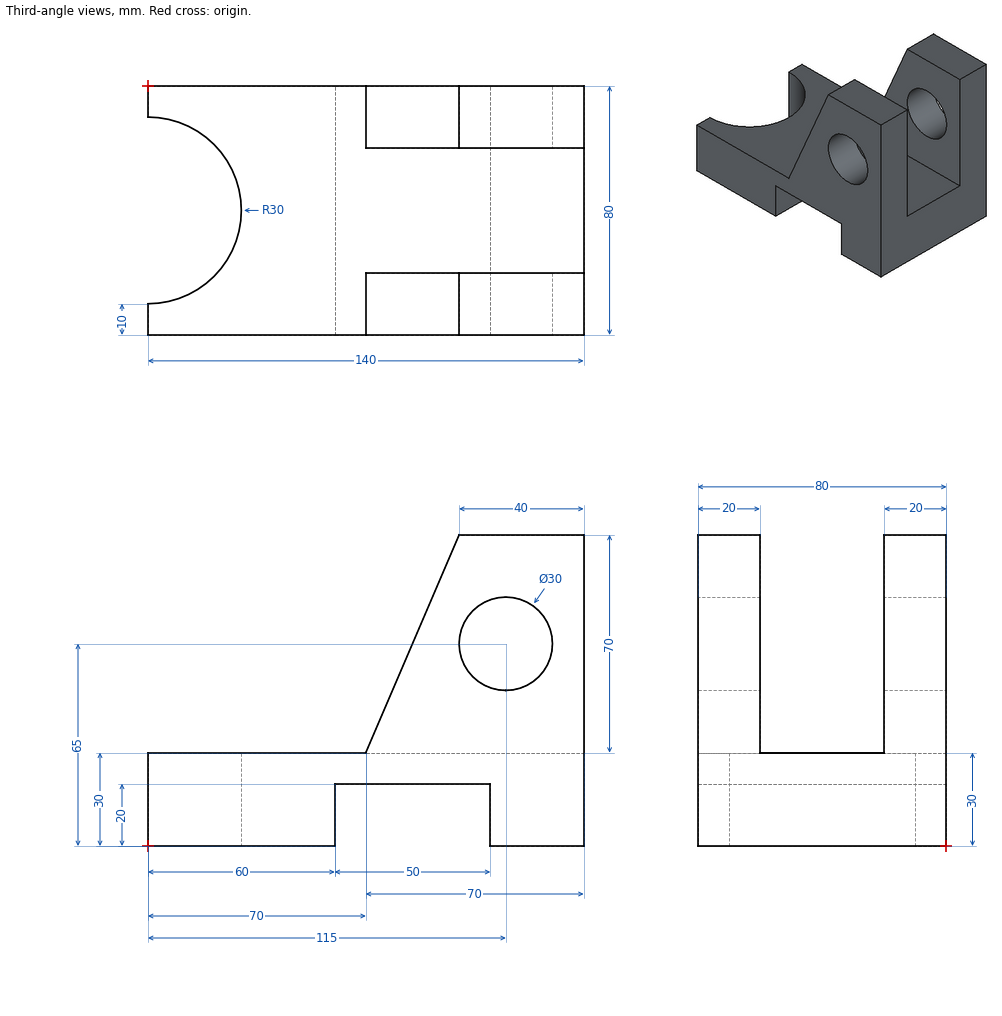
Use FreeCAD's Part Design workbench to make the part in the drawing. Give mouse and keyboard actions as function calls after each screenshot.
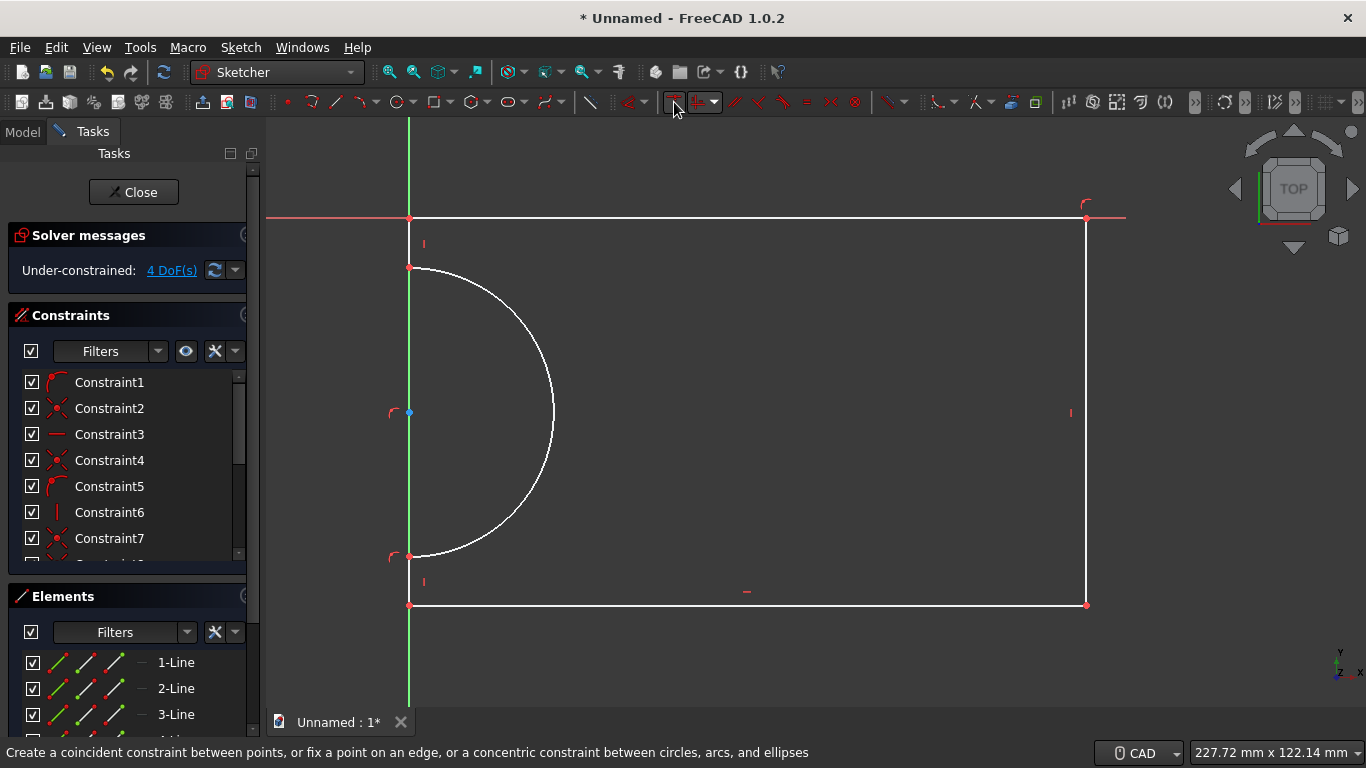
click(628, 102)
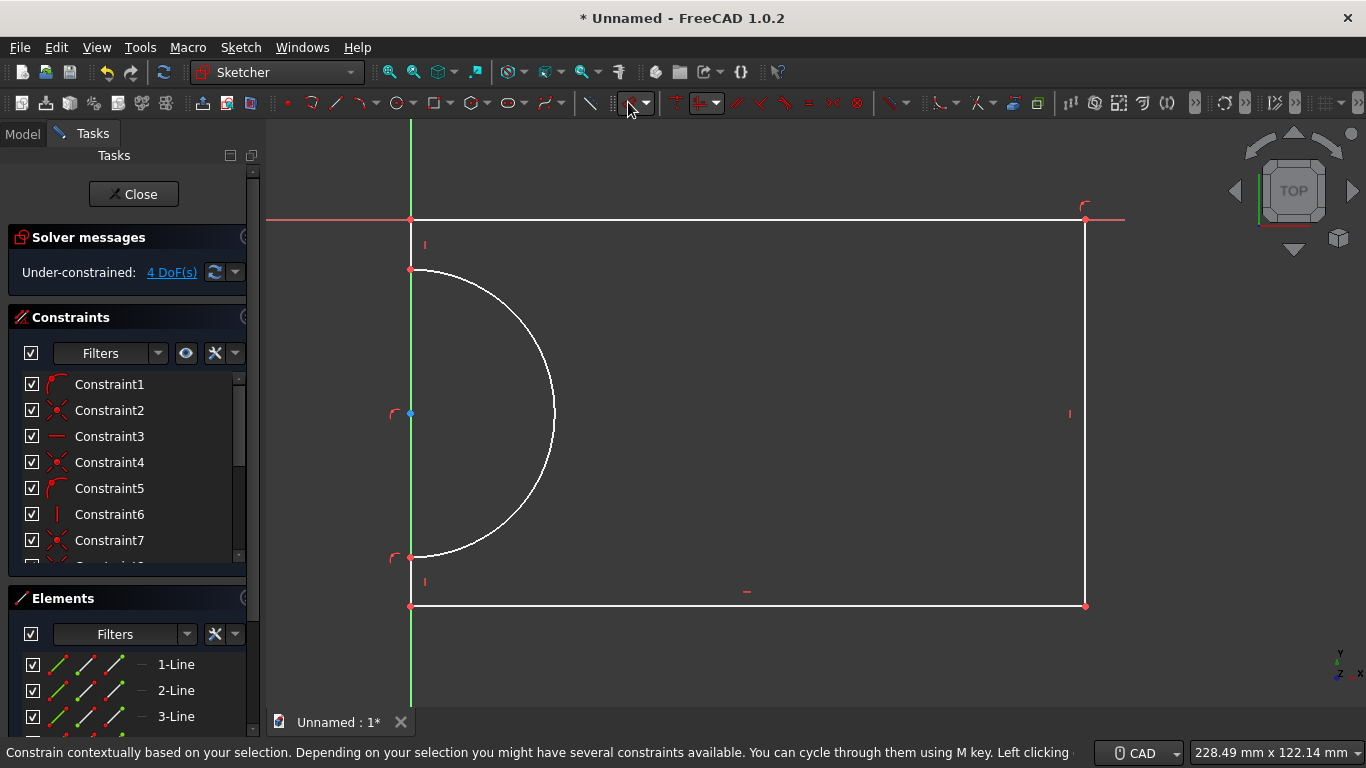
click(527, 498)
click(553, 517)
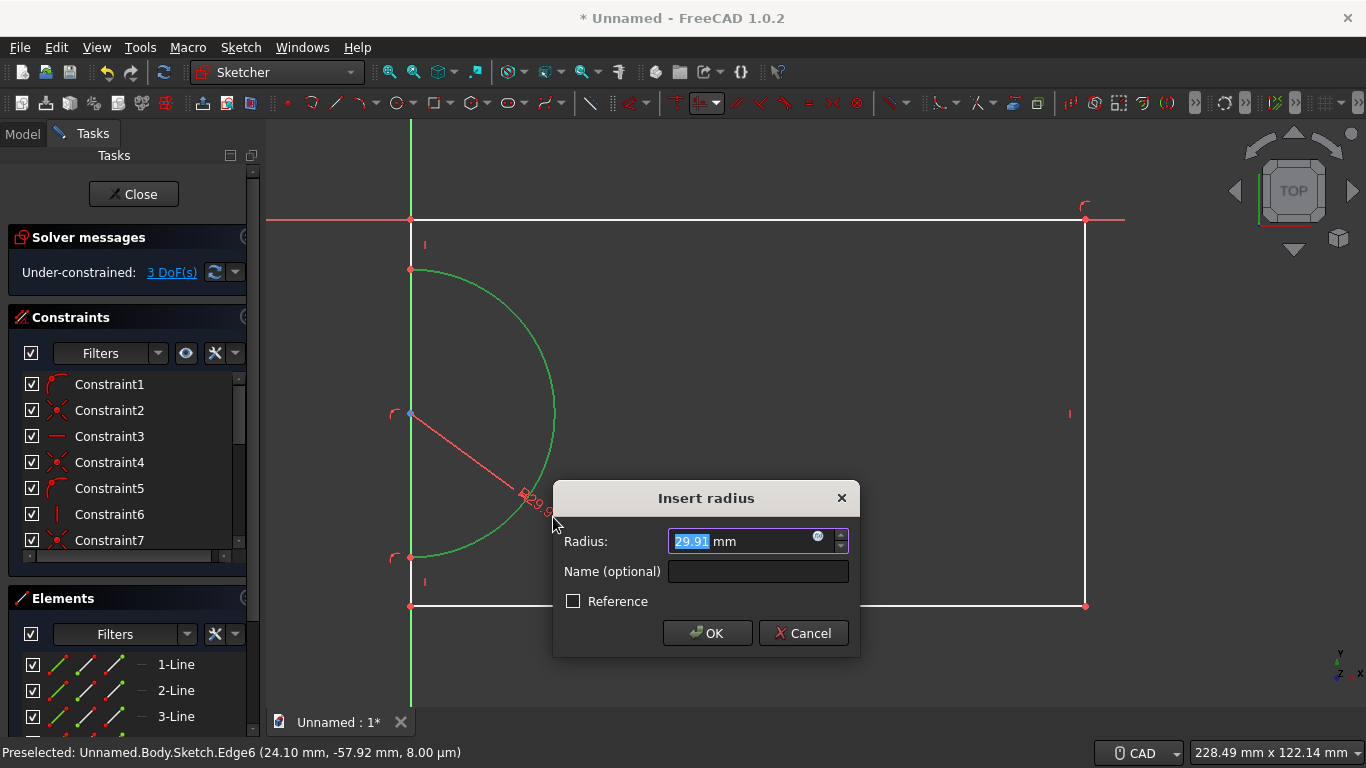
text(30)
key(Return)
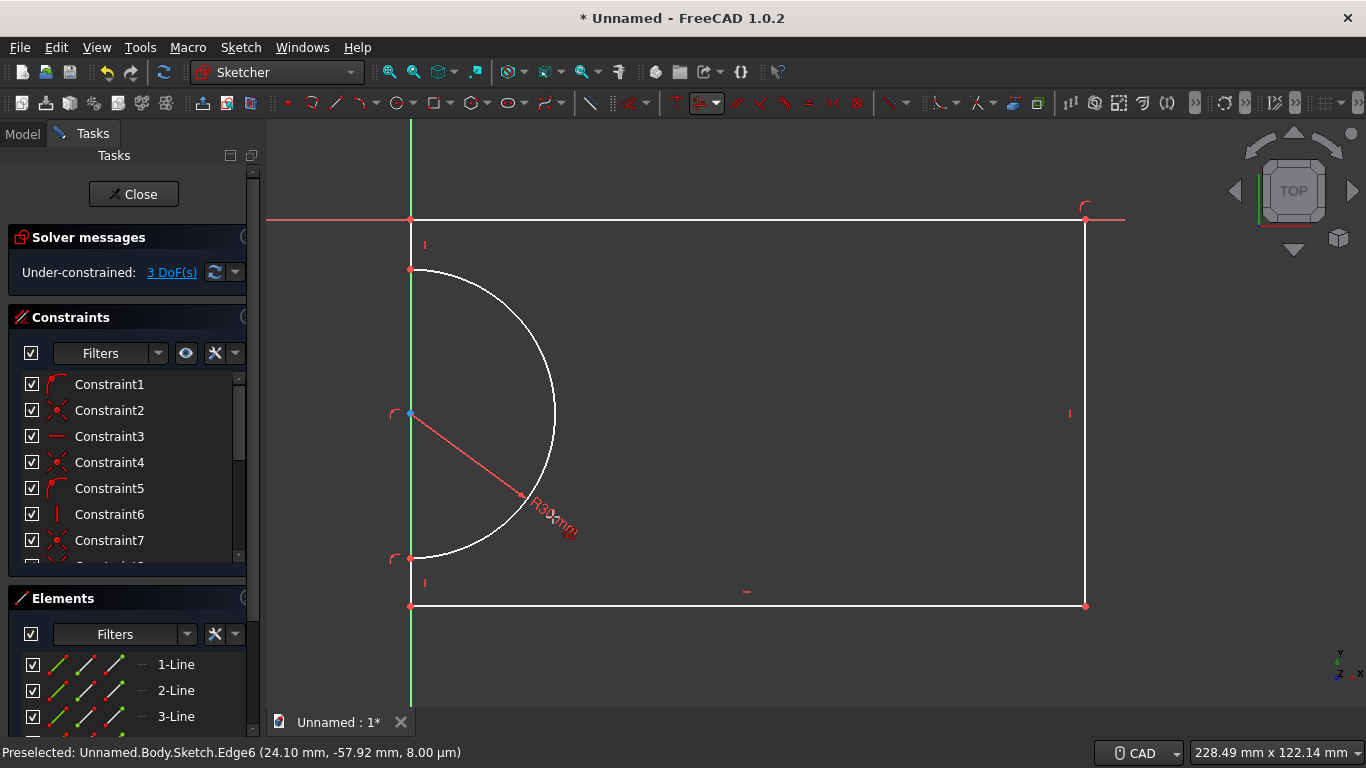
click(411, 573)
click(377, 582)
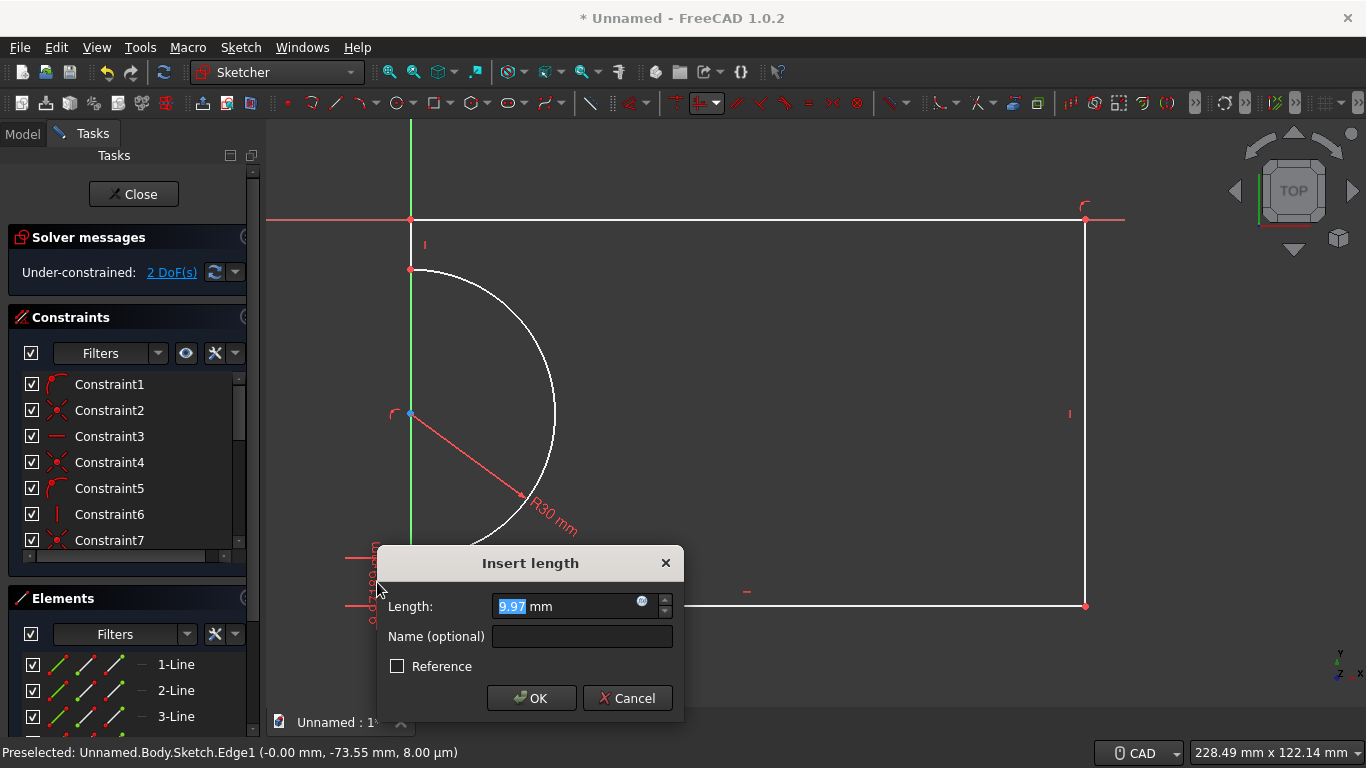
text(10)
key(Return)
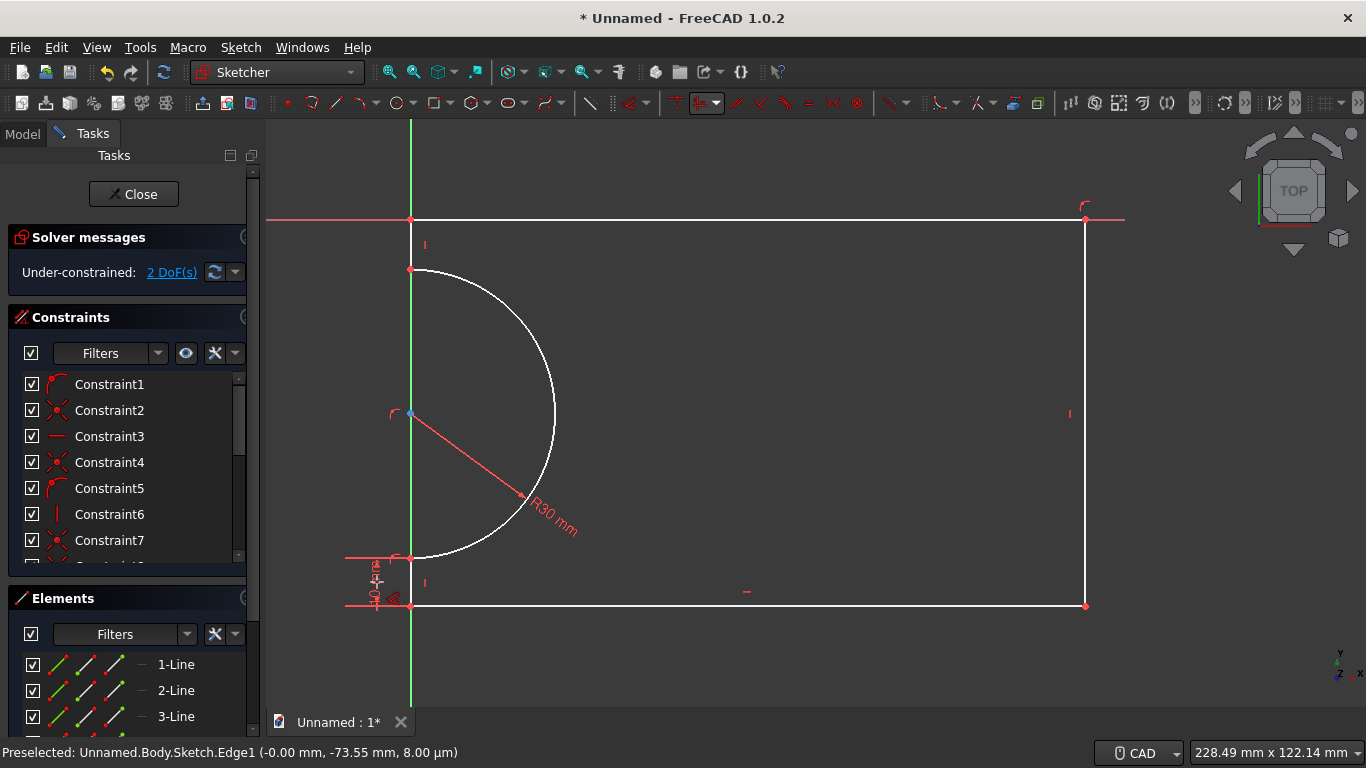
click(1085, 491)
click(1119, 413)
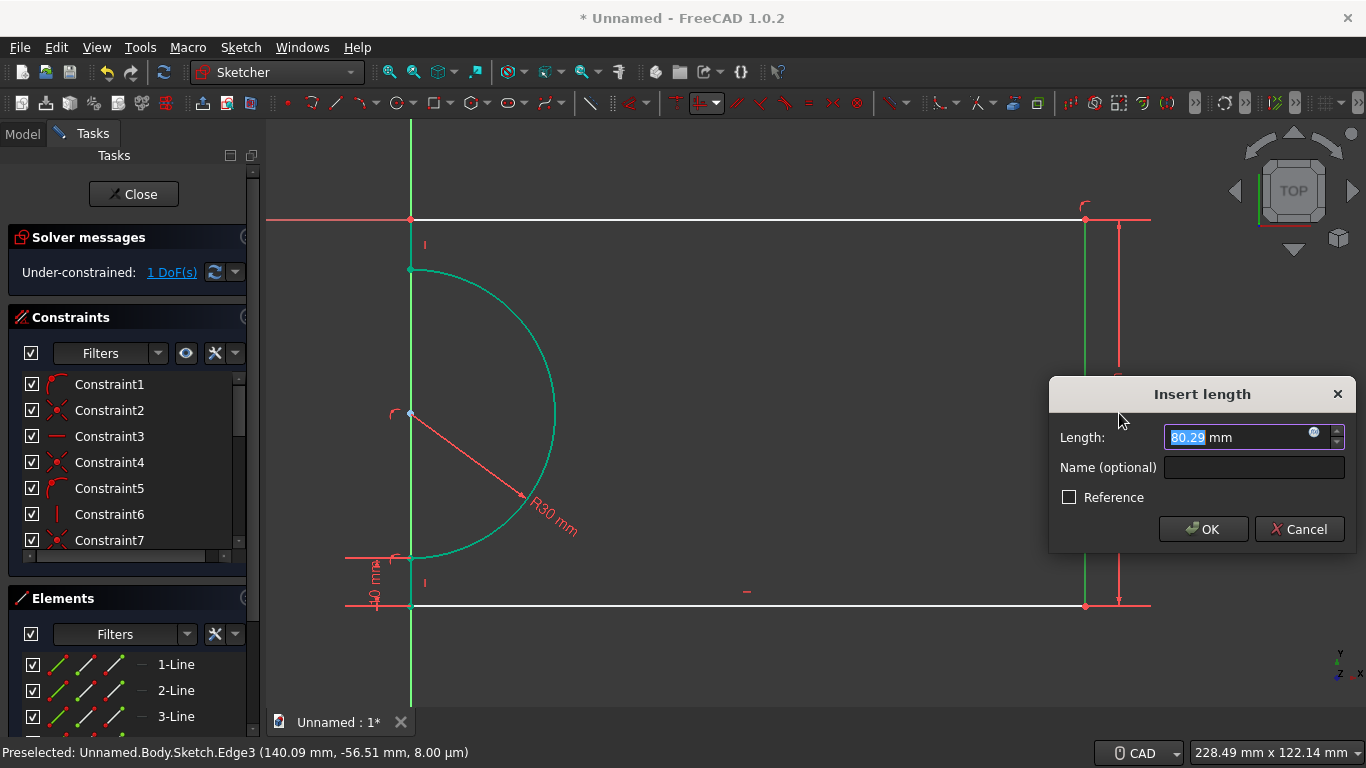
text(80)
key(Return)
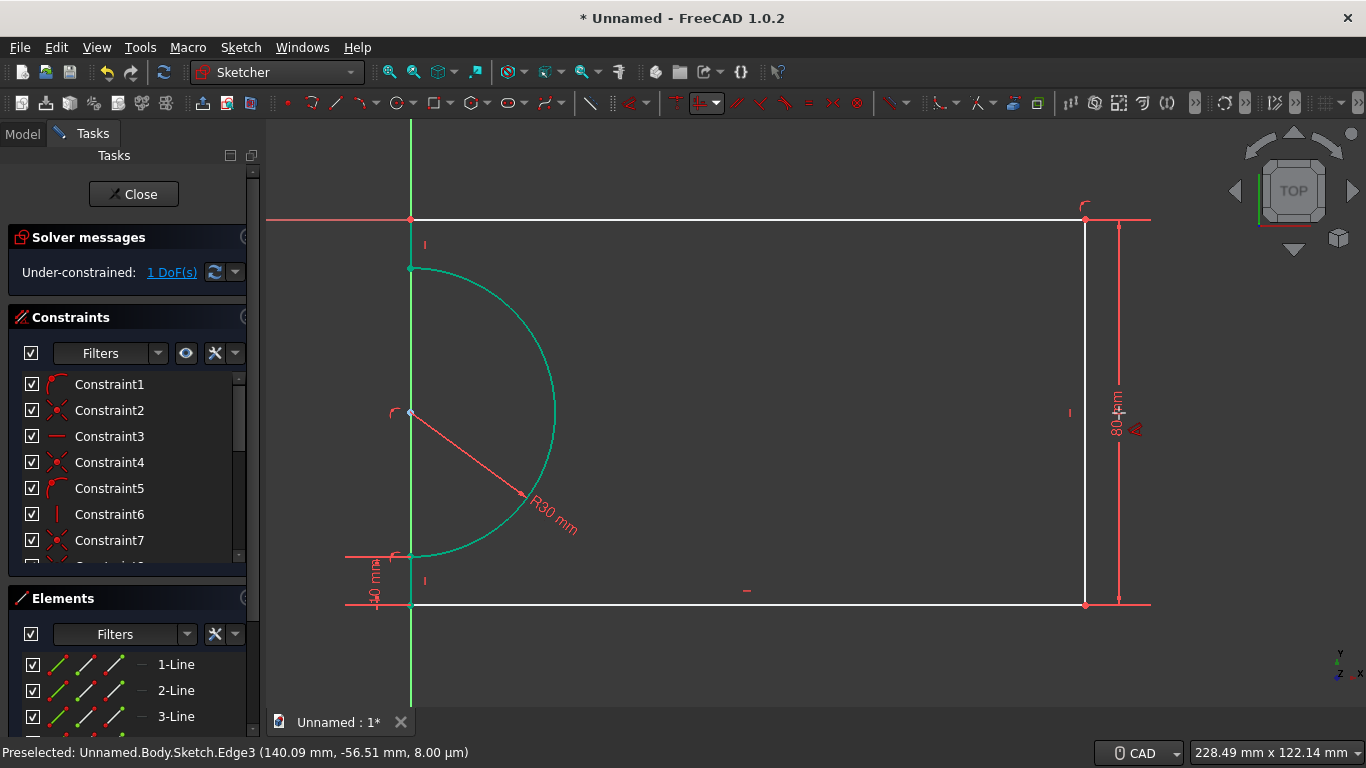
click(613, 605)
click(748, 639)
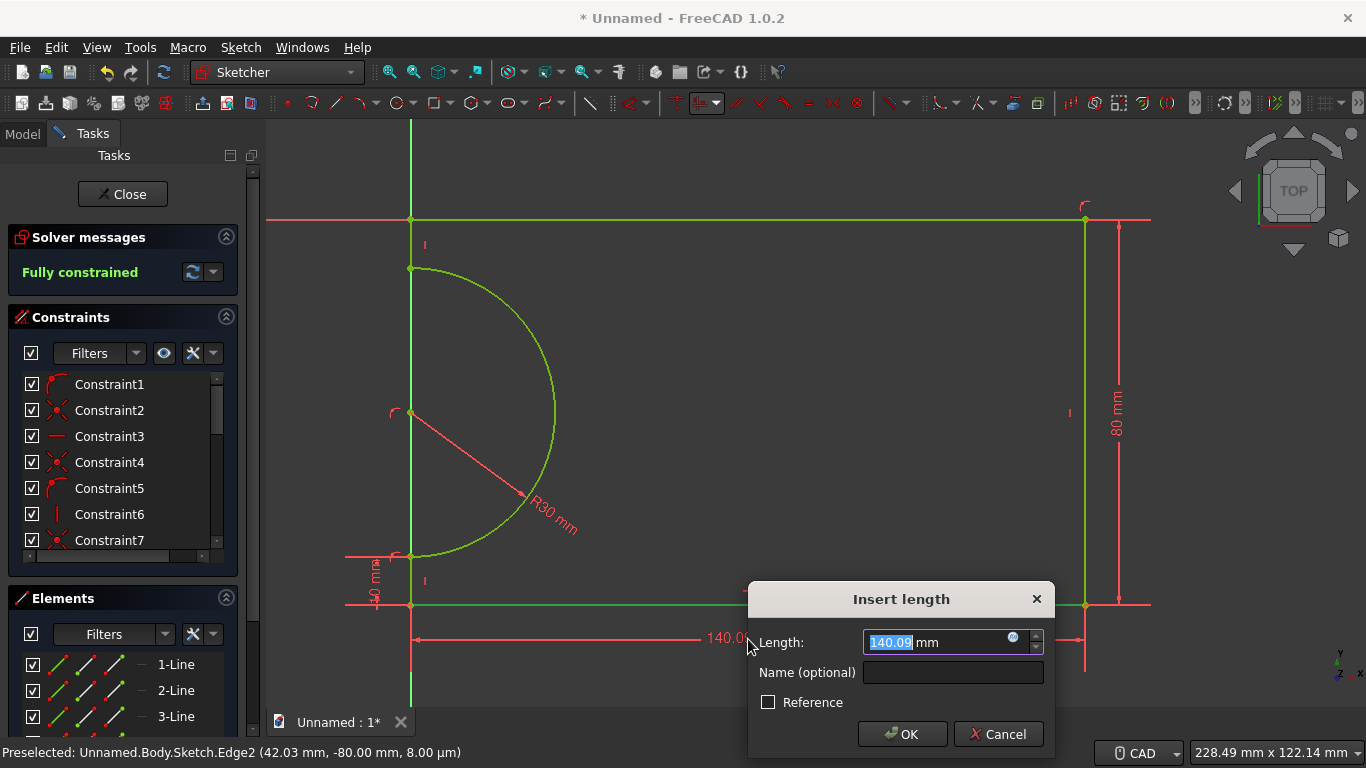
text(140)
key(Return)
key(Escape)